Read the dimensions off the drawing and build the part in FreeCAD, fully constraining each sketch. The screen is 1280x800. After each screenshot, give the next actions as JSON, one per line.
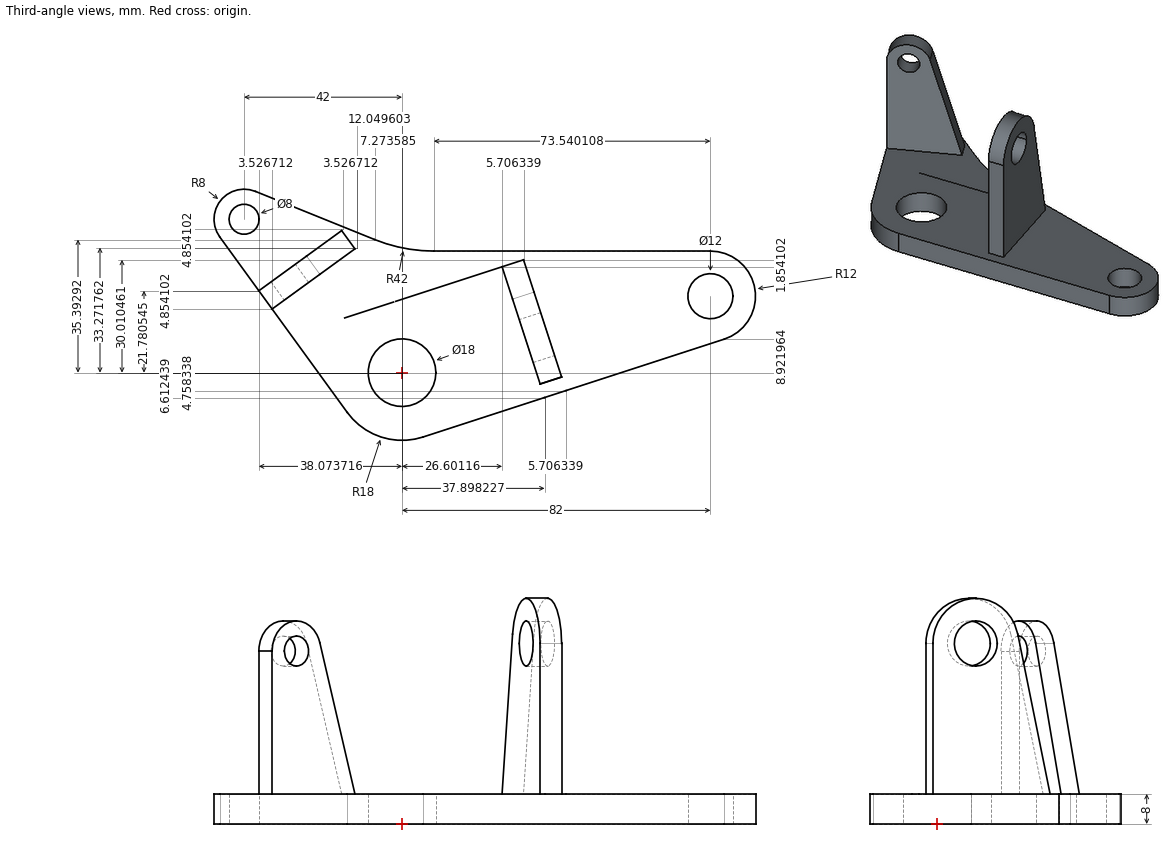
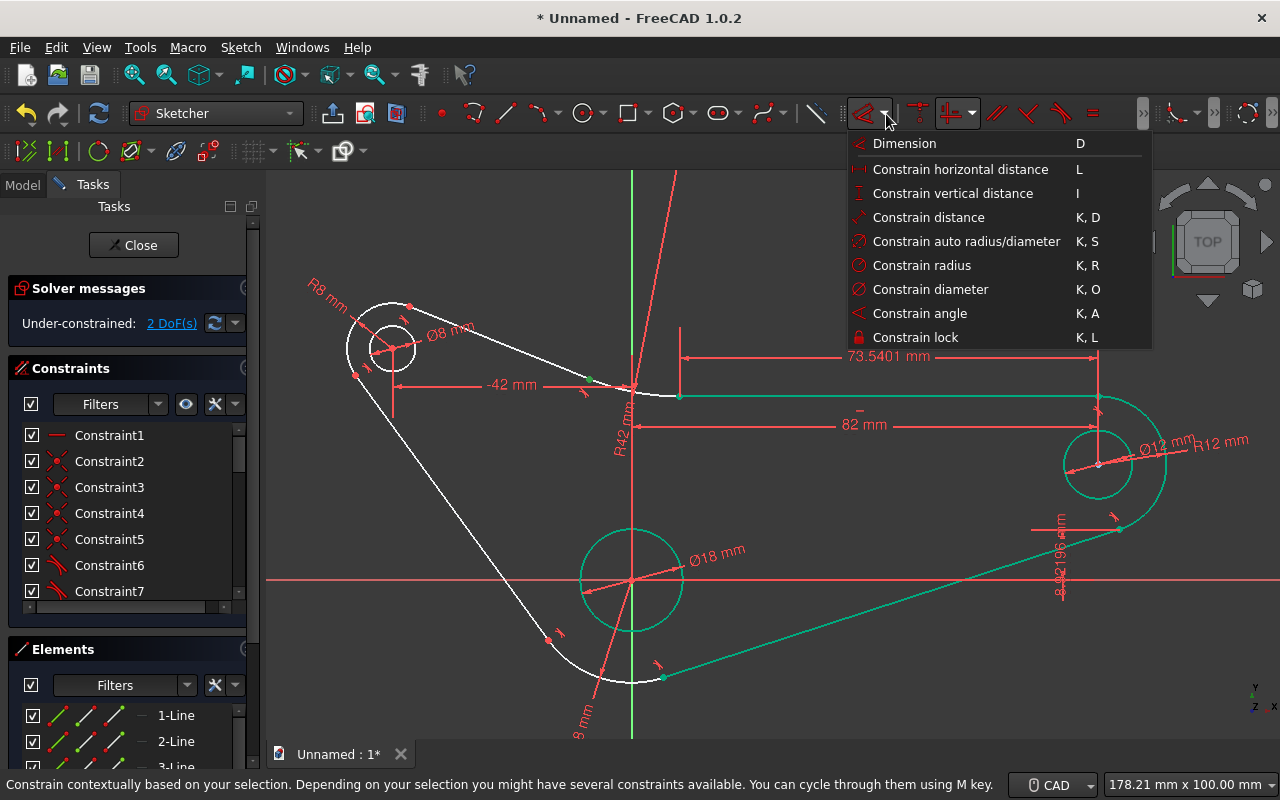
{"action": "left_click", "coordinate": [1000, 169]}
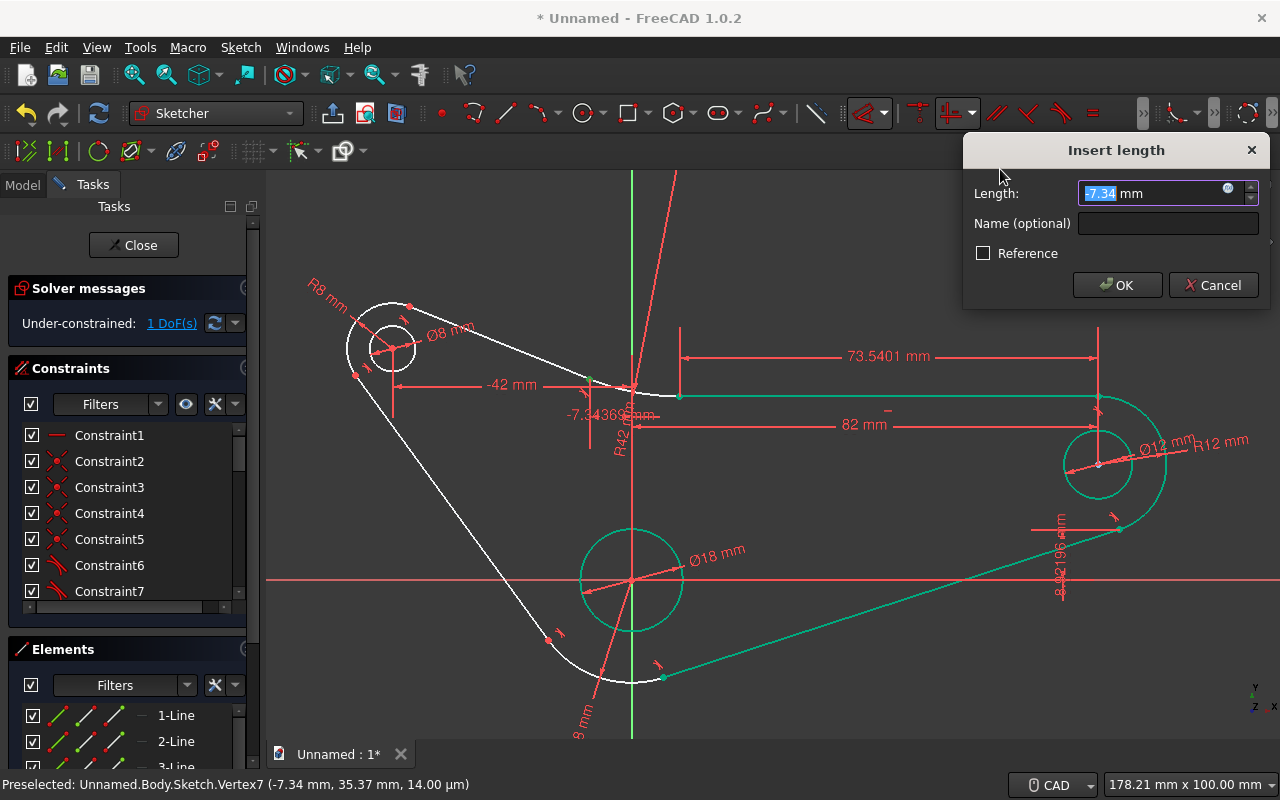
{"action": "type", "text": "-7.273585"}
{"action": "key", "text": "Return"}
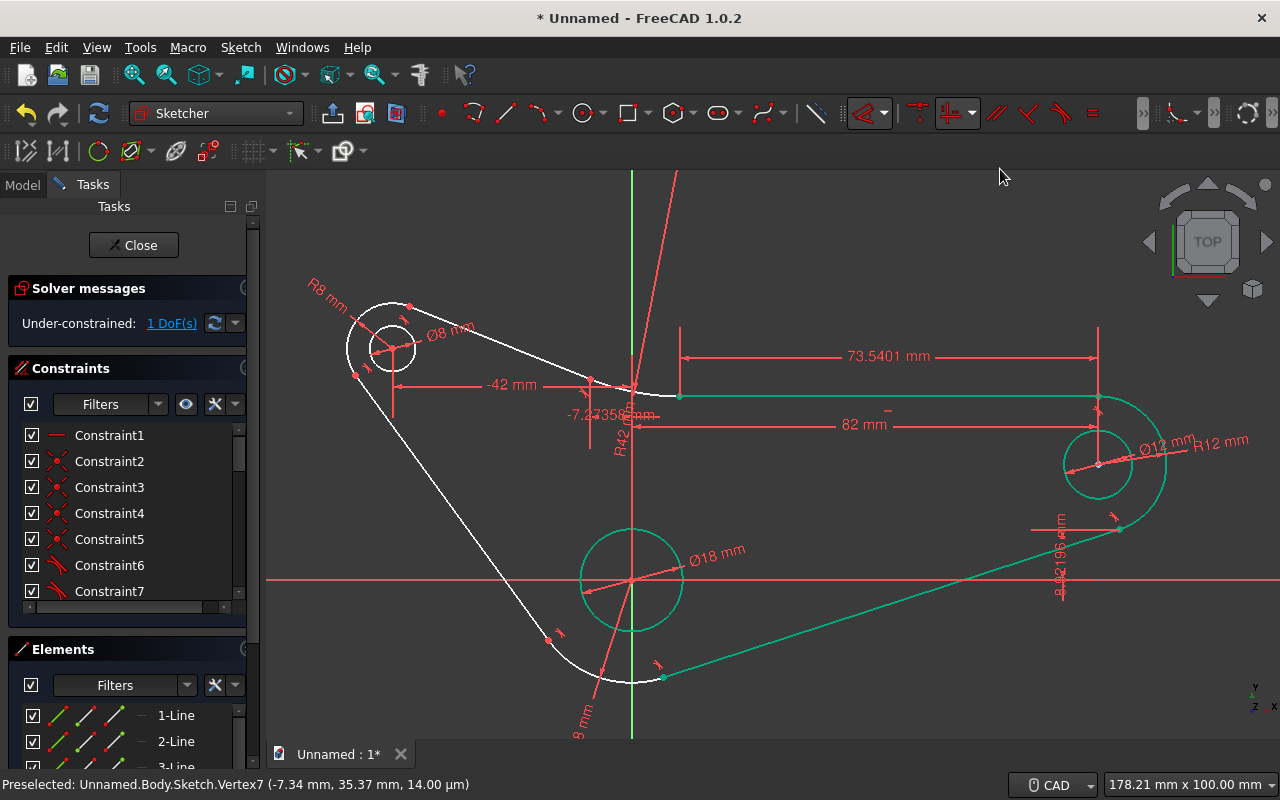
{"action": "left_click", "coordinate": [590, 379]}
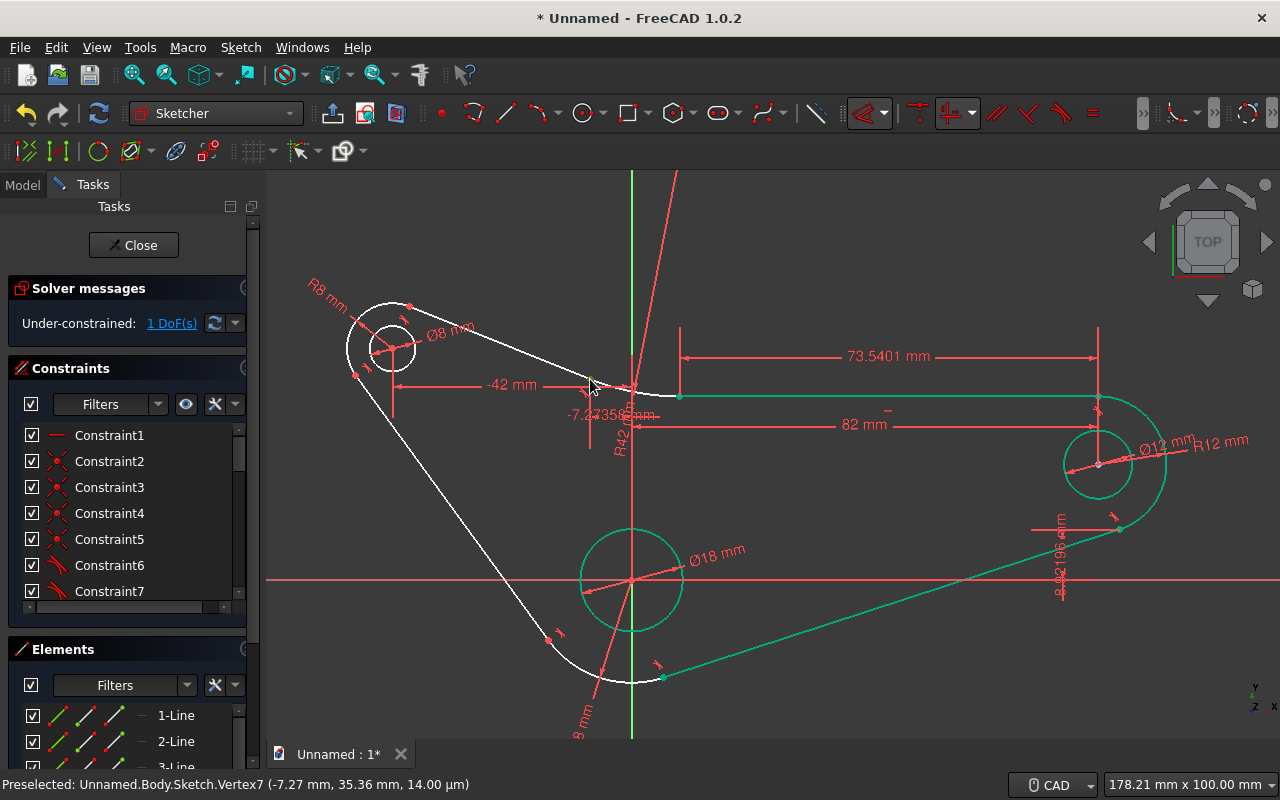
{"action": "key", "text": "i"}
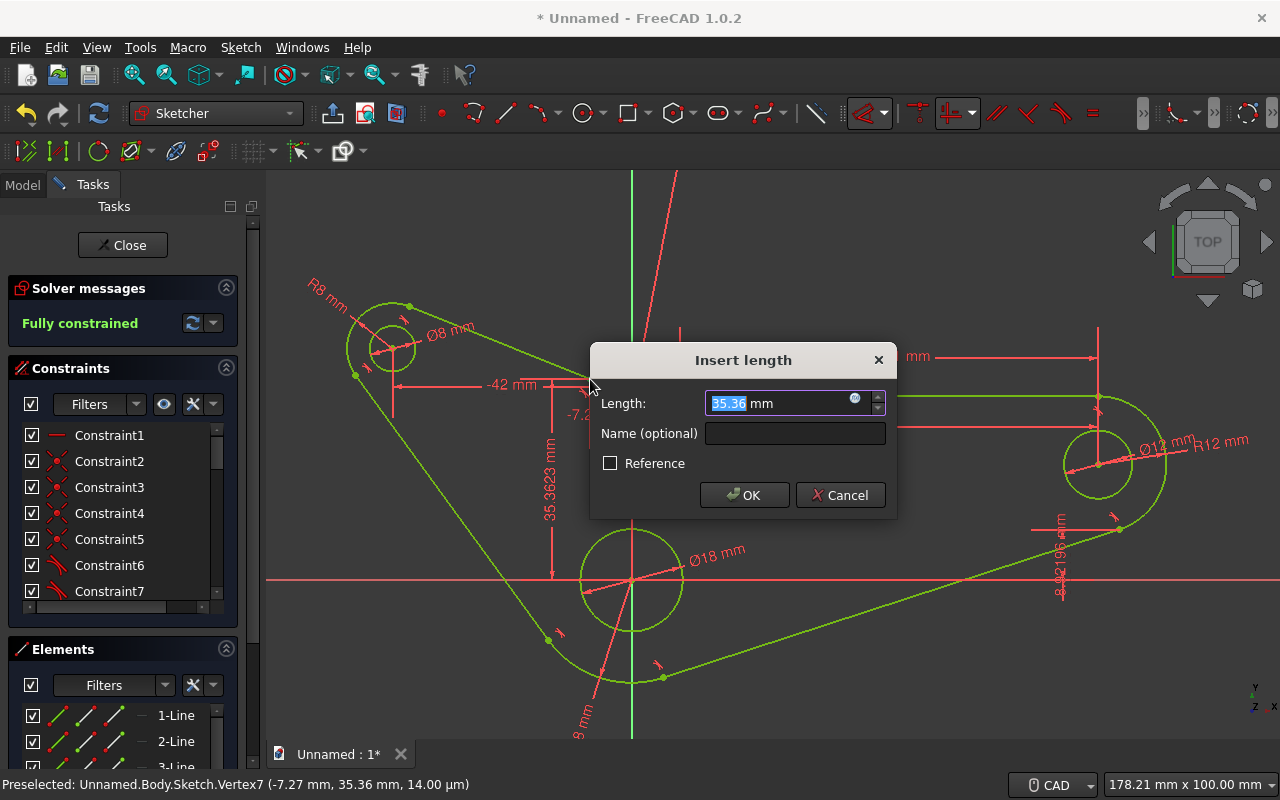
{"action": "type", "text": "35.39292"}
{"action": "key", "text": "Return"}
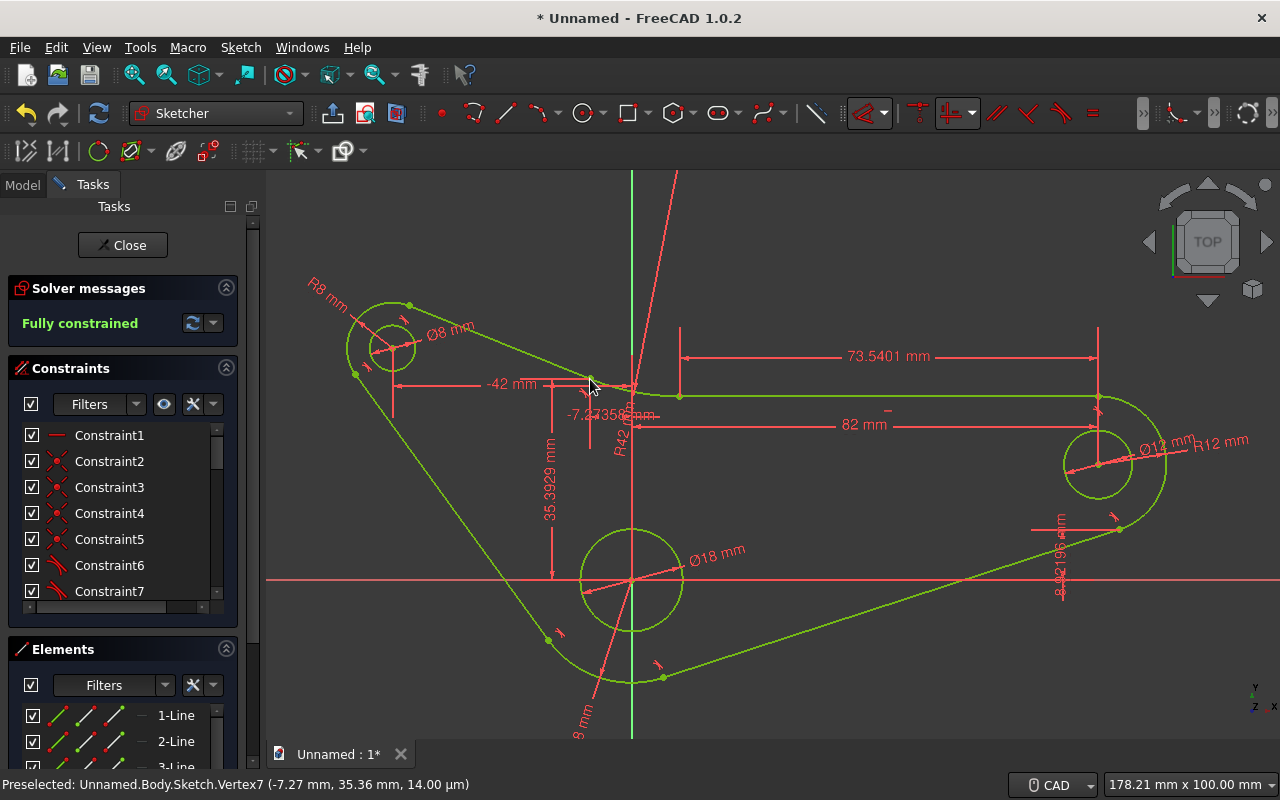
{"action": "left_click", "coordinate": [123, 245]}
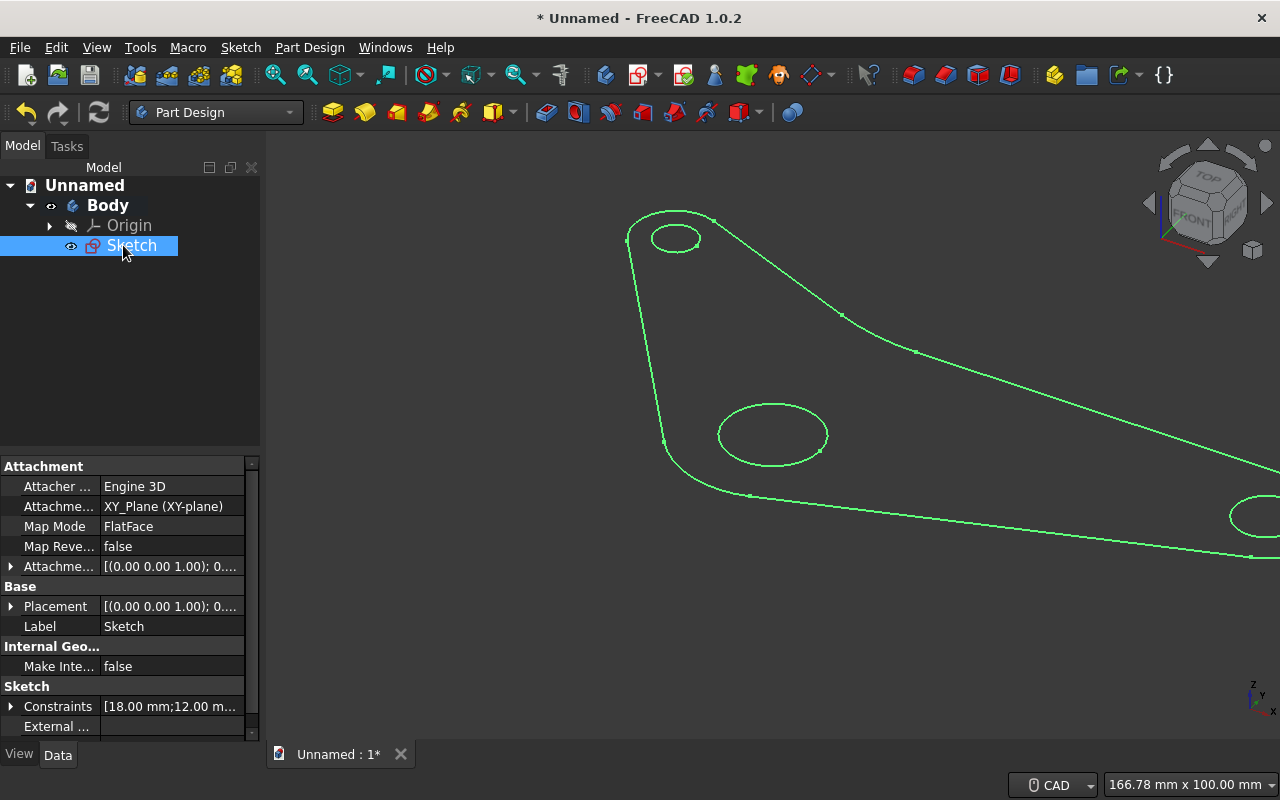
{"action": "left_click", "coordinate": [334, 112]}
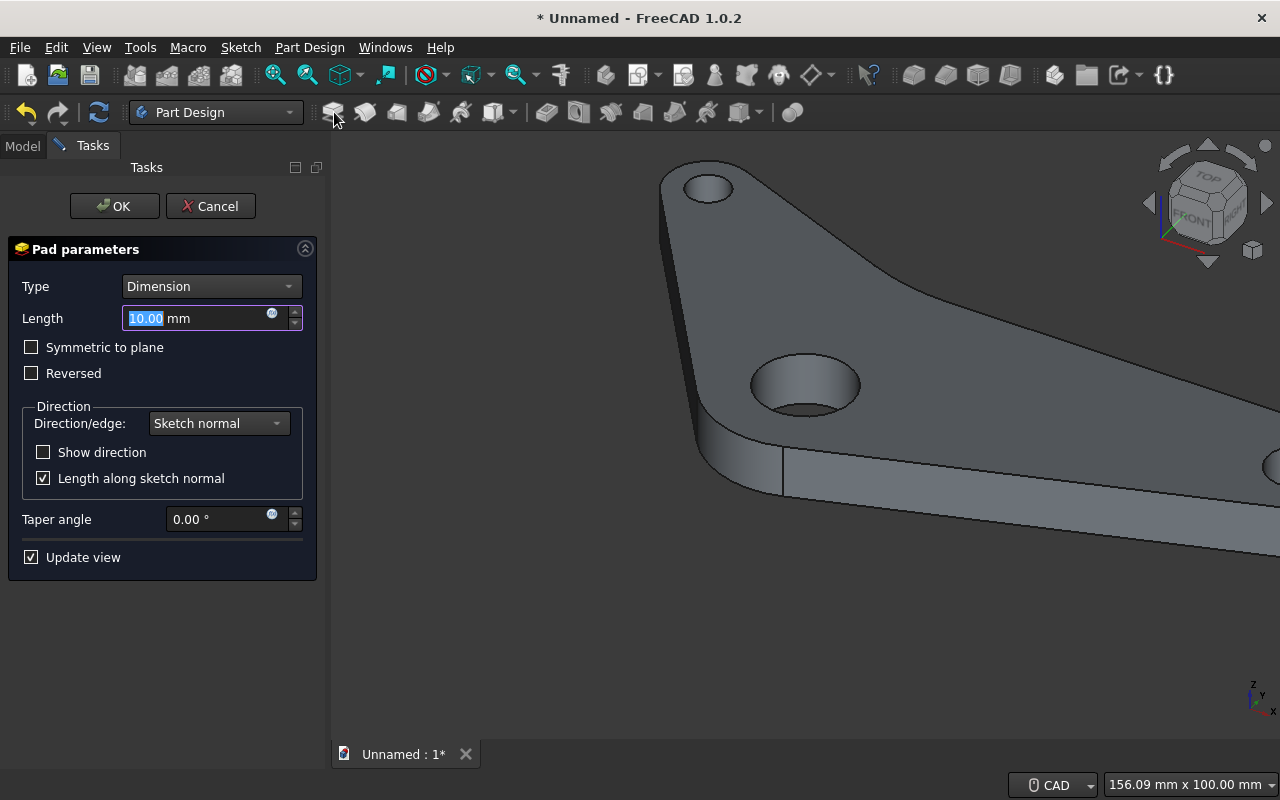
{"action": "type", "text": "8"}
{"action": "key", "text": "Tab"}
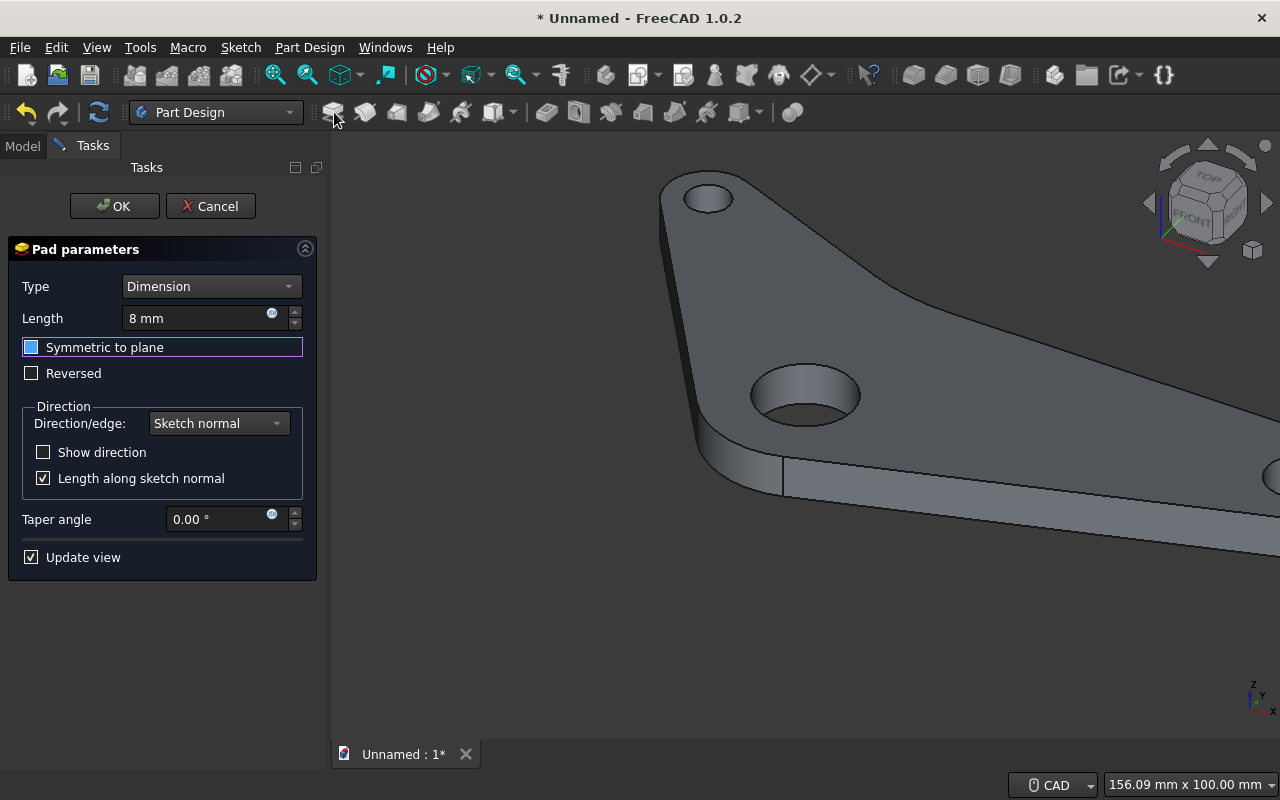
{"action": "left_click", "coordinate": [115, 206]}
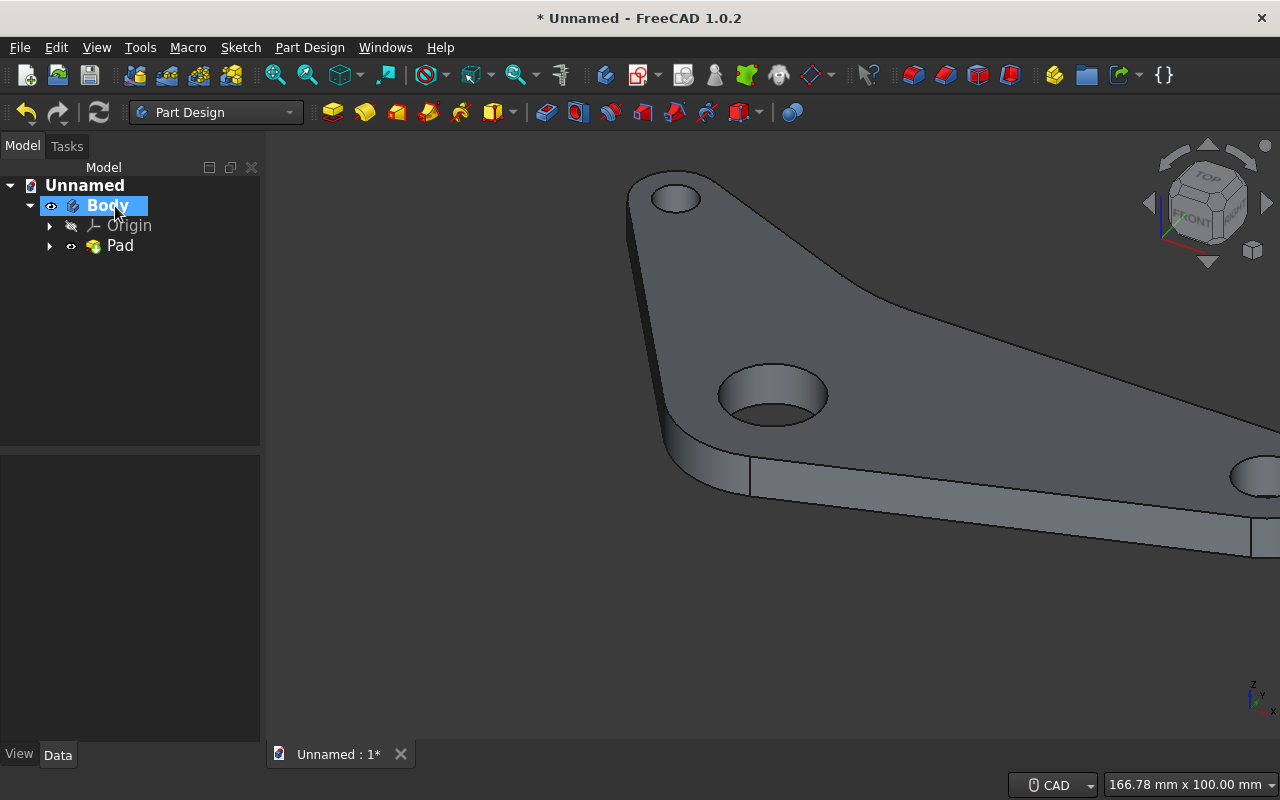
{"action": "key", "text": "v f"}